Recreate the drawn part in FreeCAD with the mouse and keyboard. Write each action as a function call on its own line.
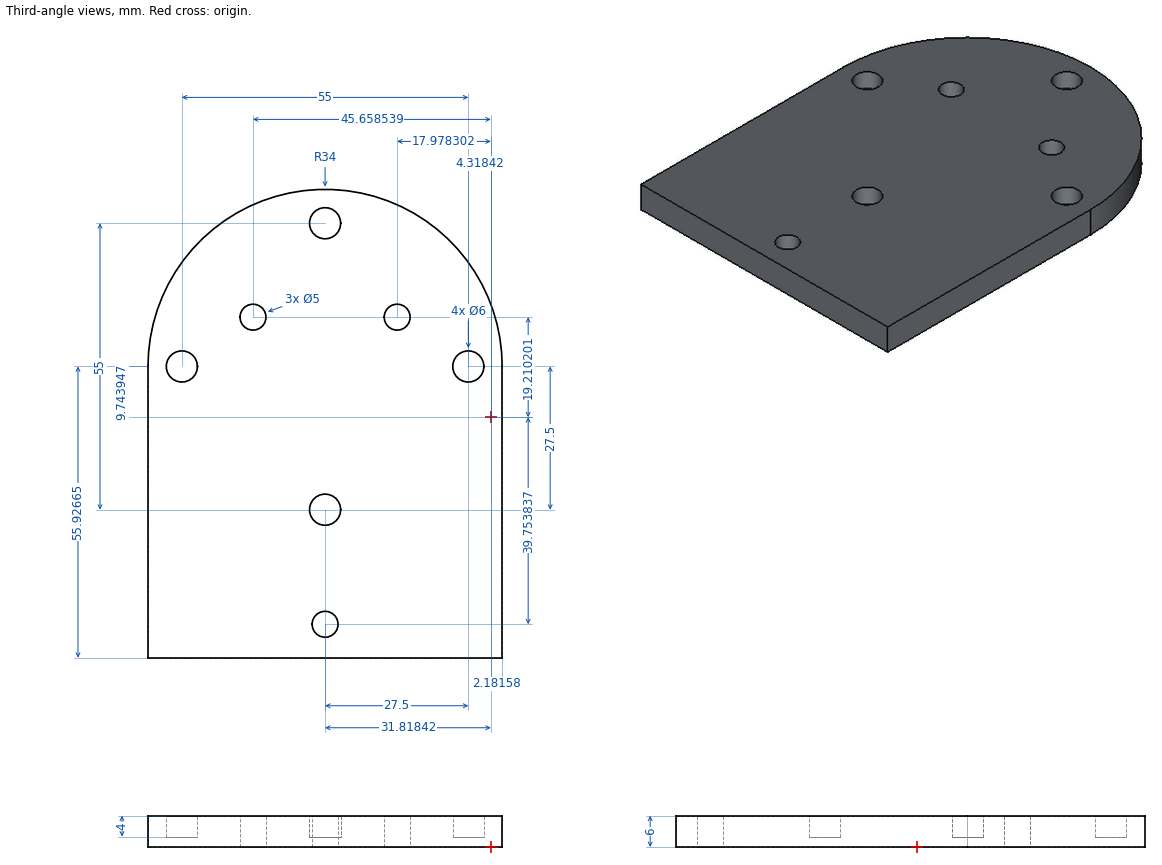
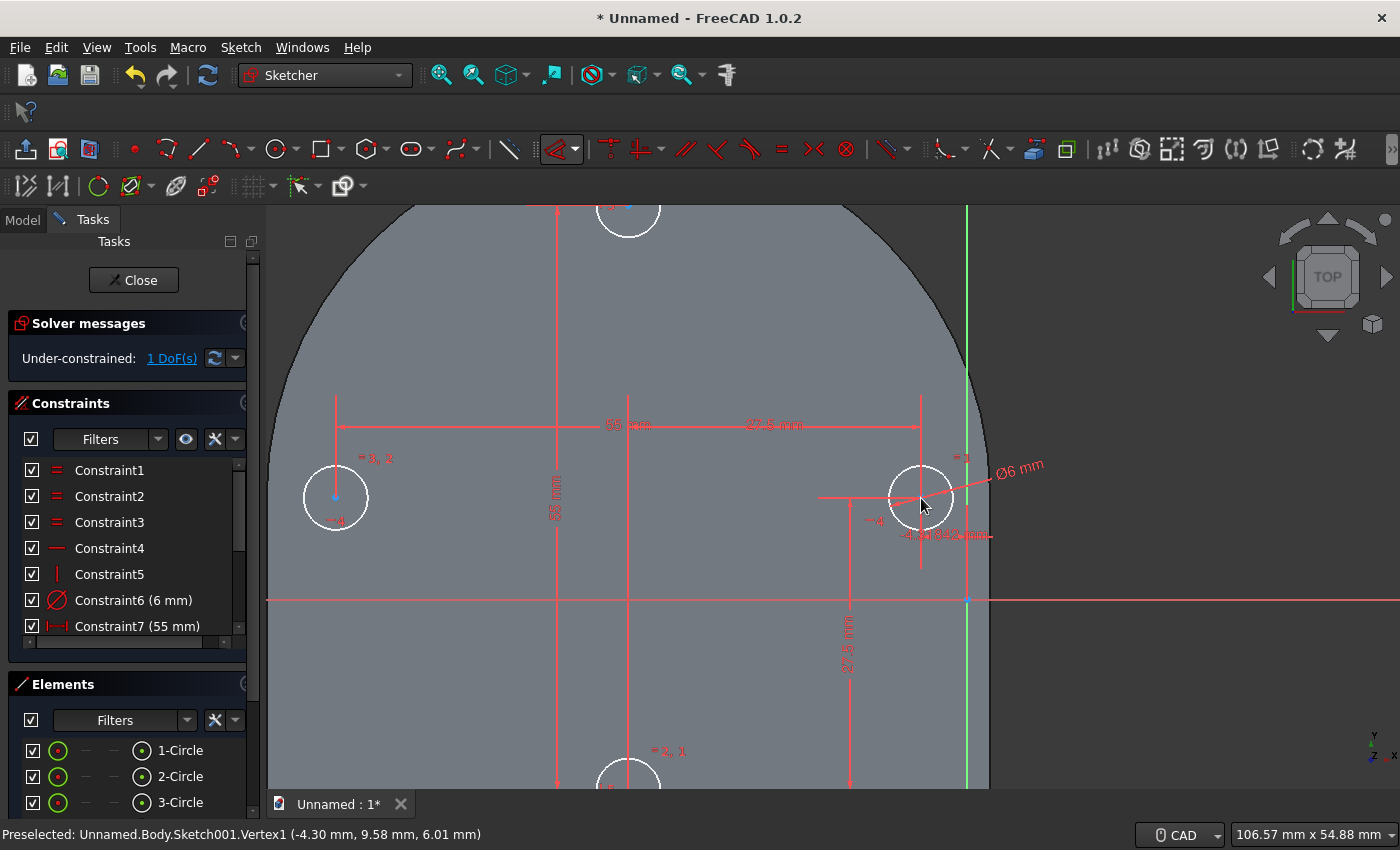
click(921, 498)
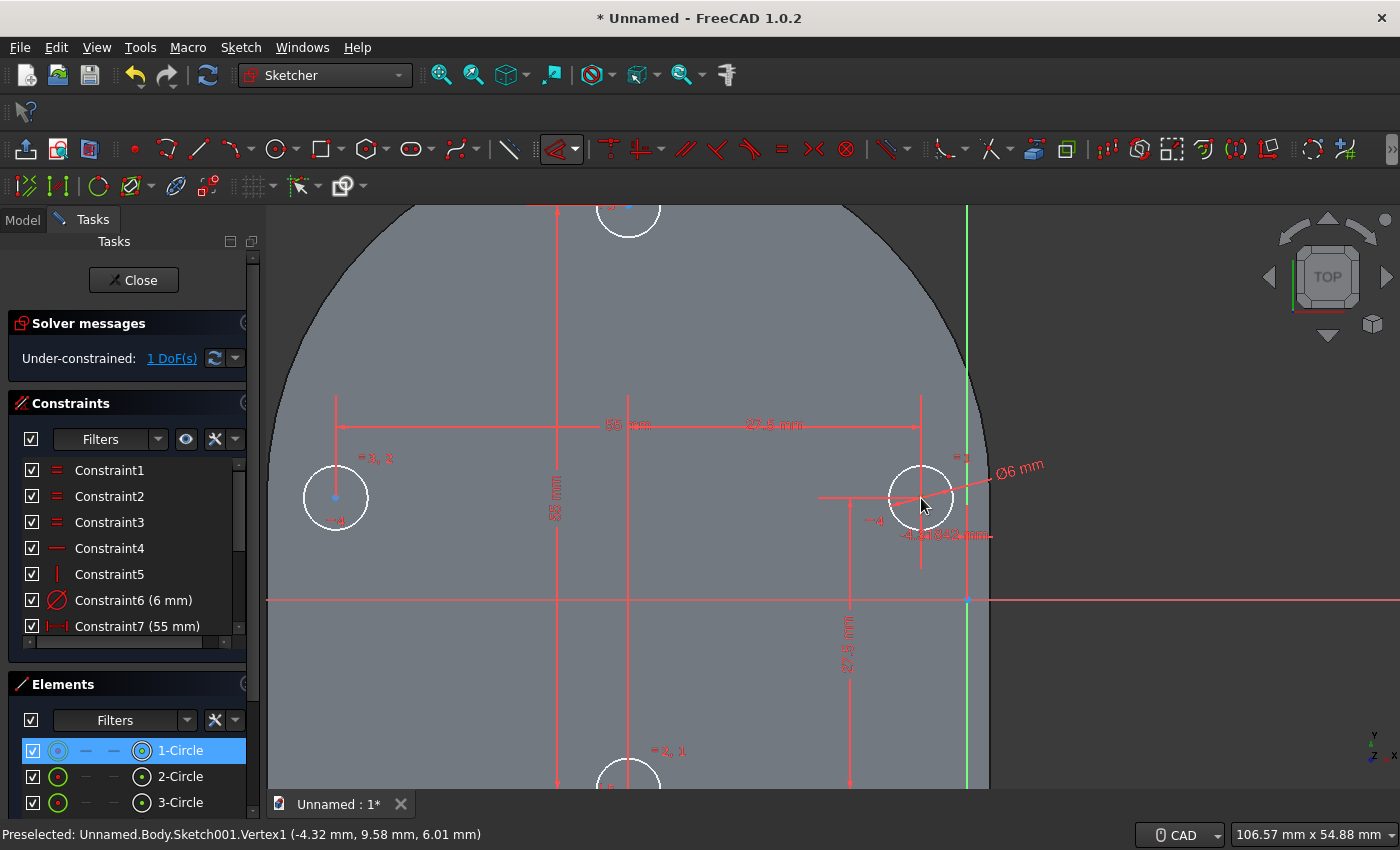
key(i)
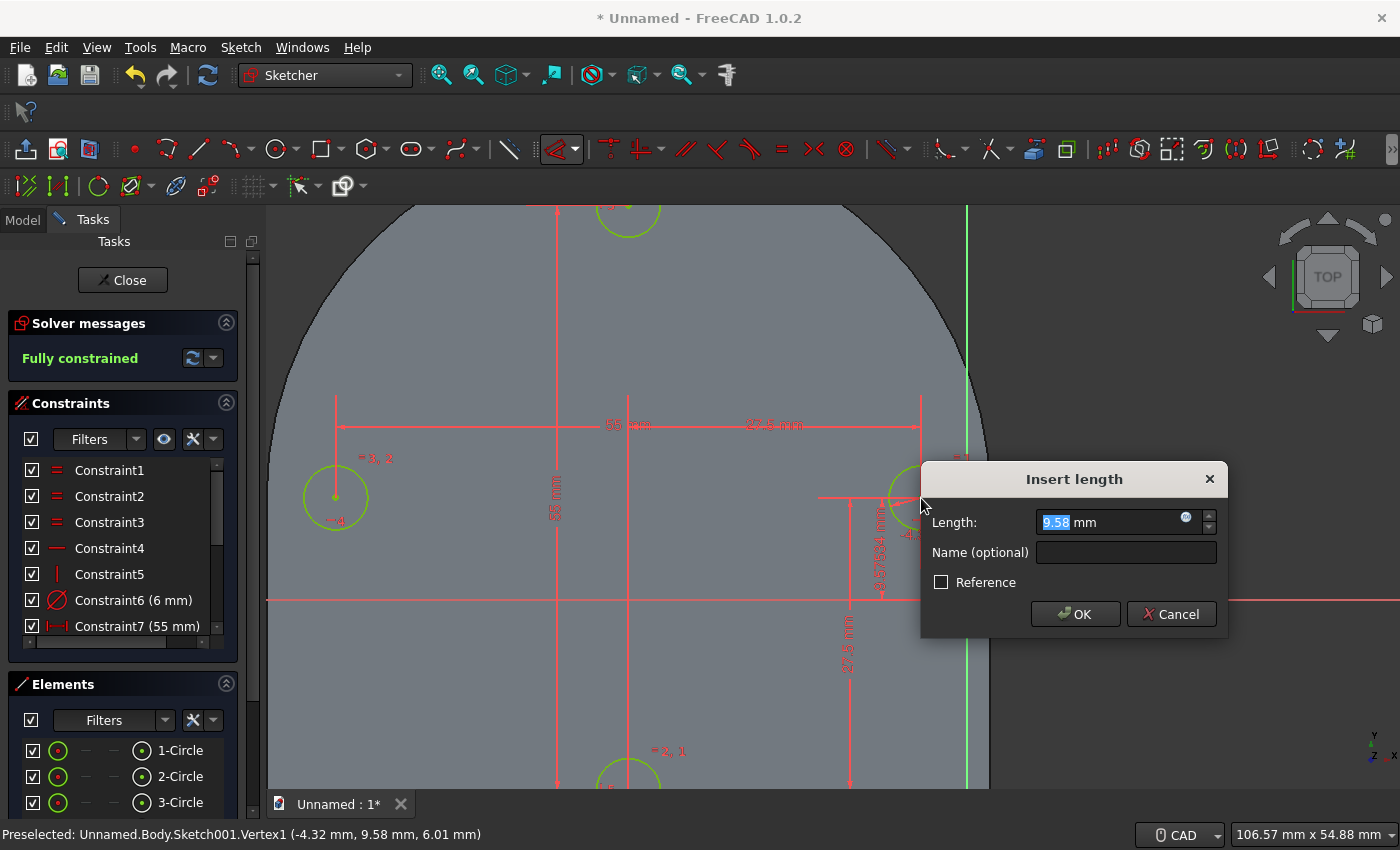
text(9.743947)
key(Return)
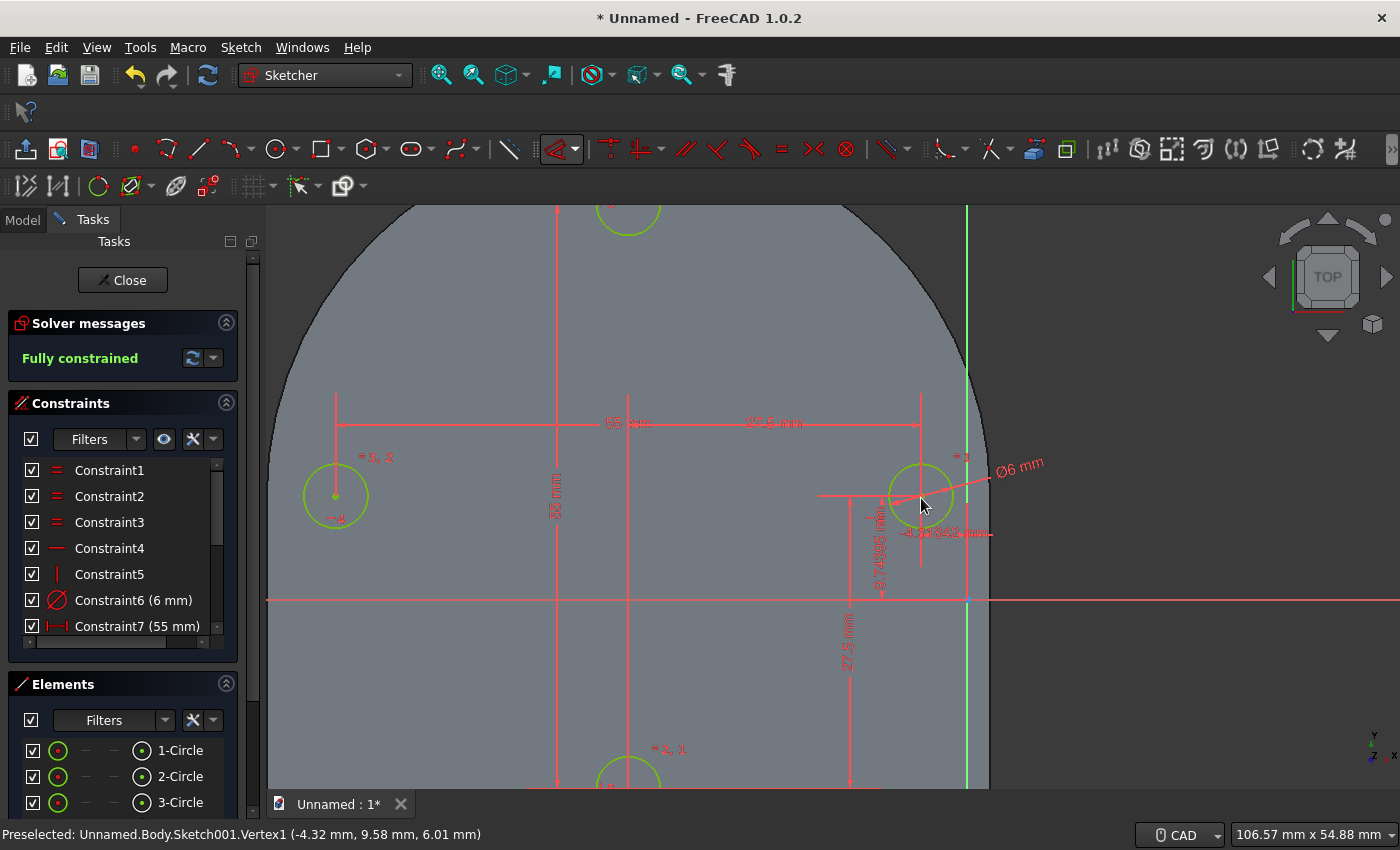
click(123, 280)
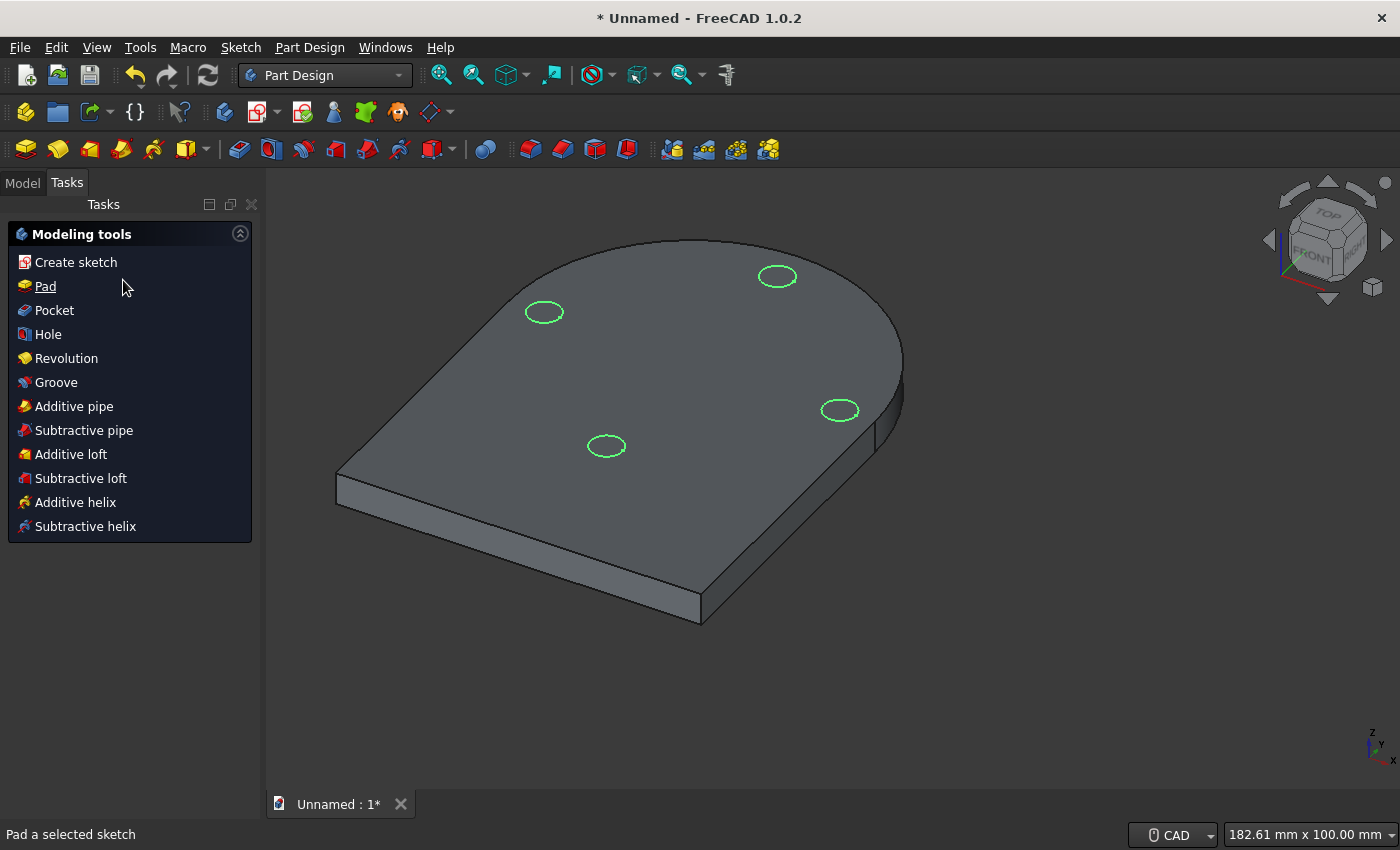
click(240, 150)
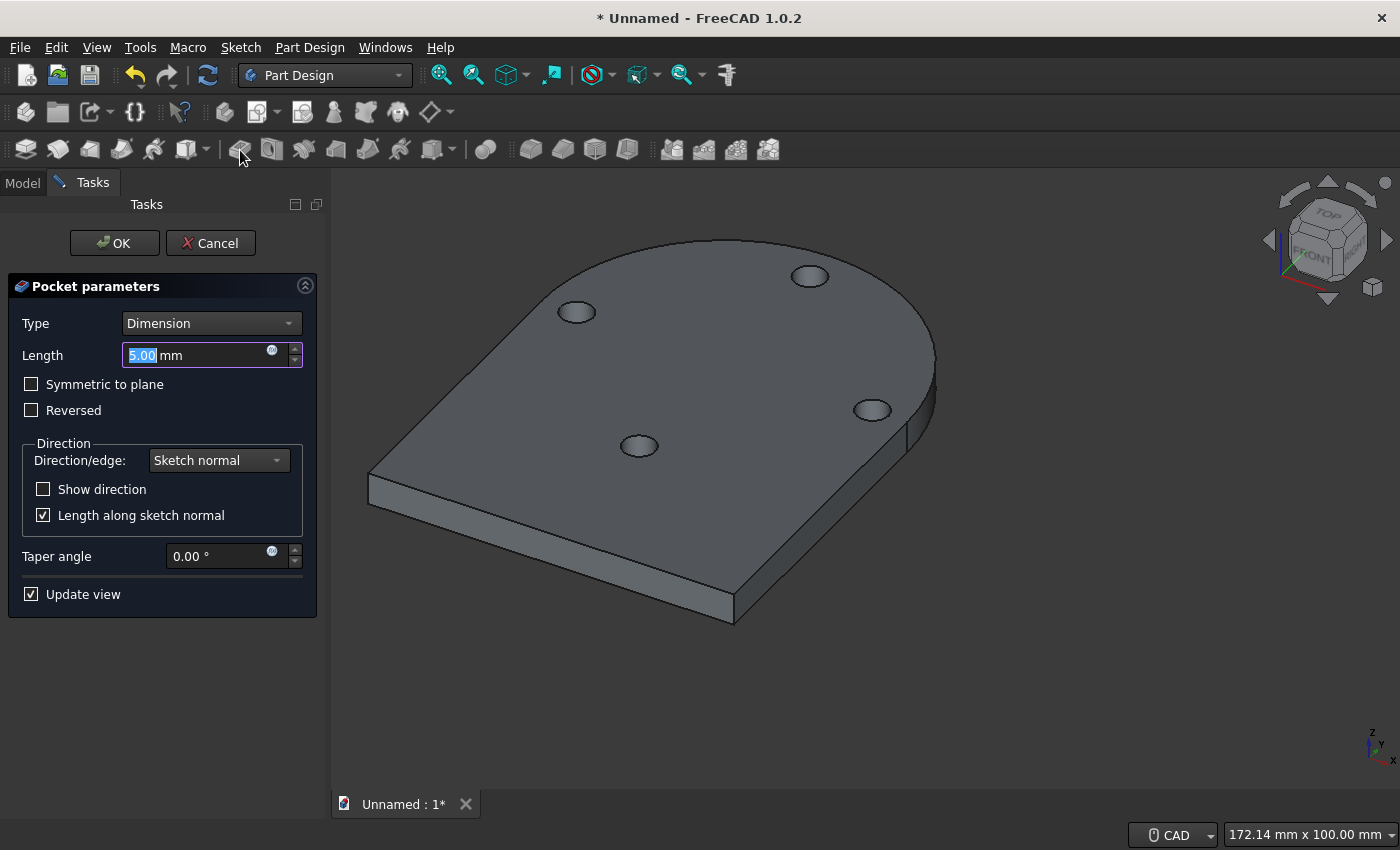
text(4)
key(Tab)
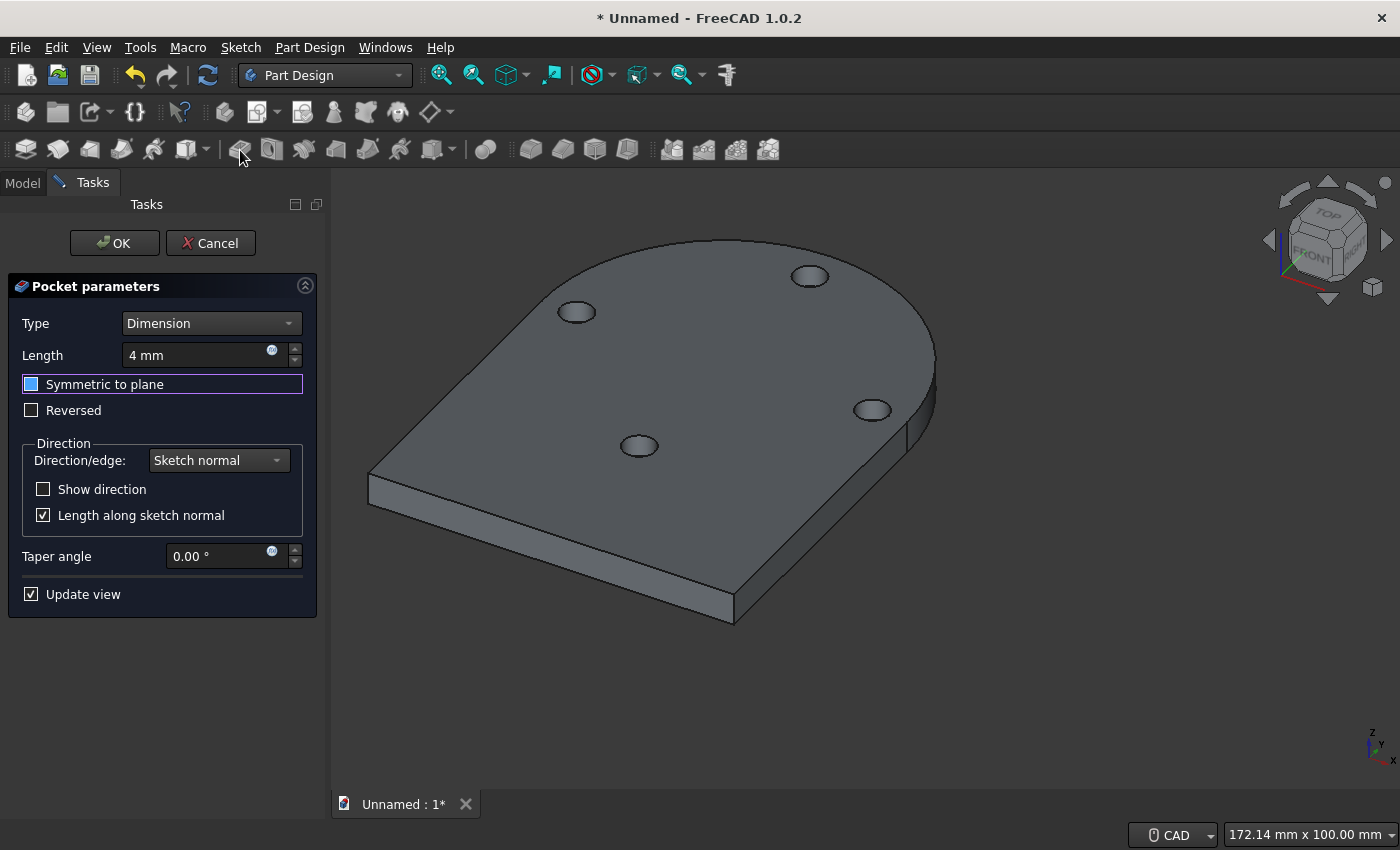
click(115, 243)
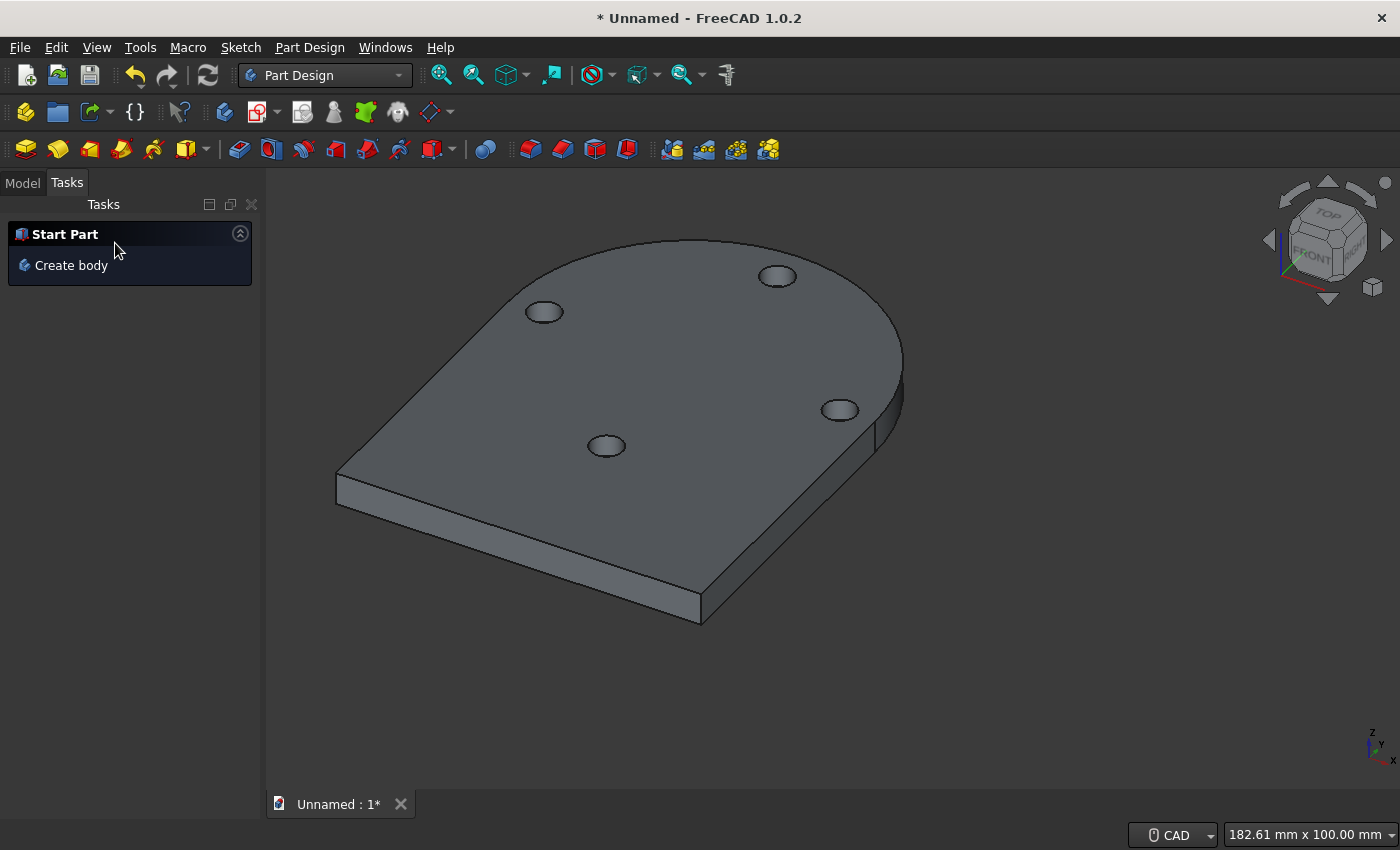
key(5)